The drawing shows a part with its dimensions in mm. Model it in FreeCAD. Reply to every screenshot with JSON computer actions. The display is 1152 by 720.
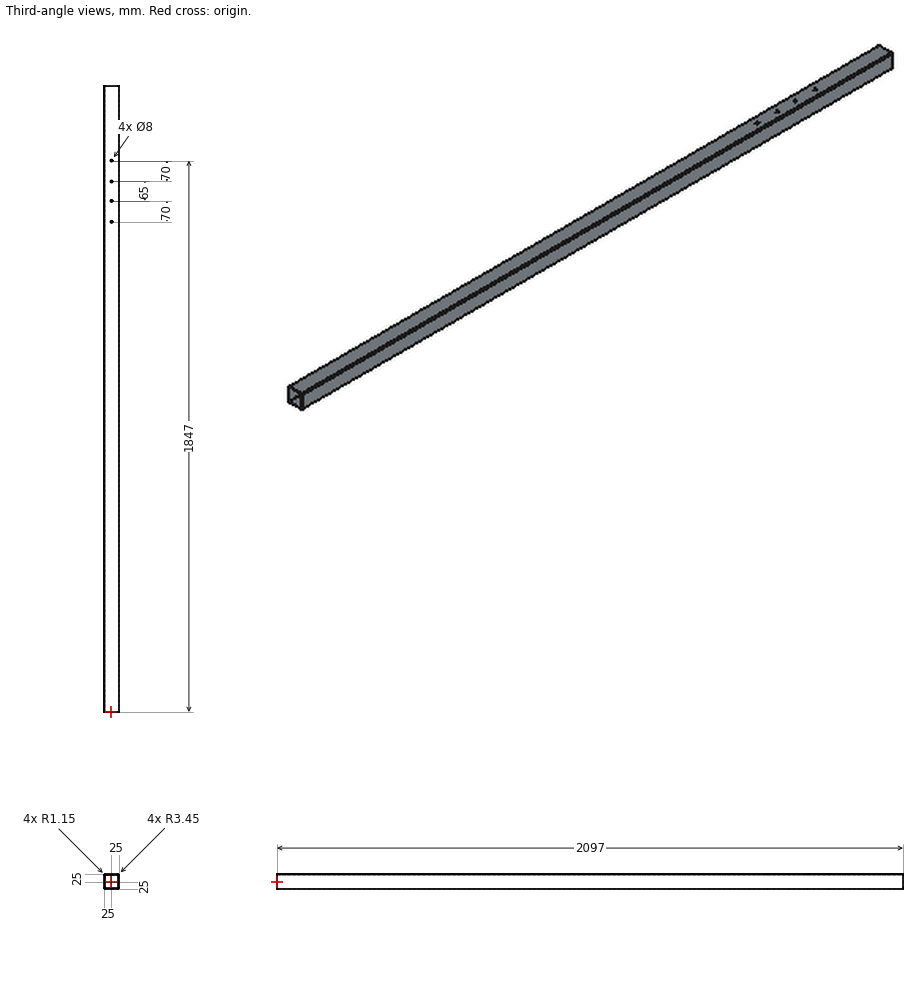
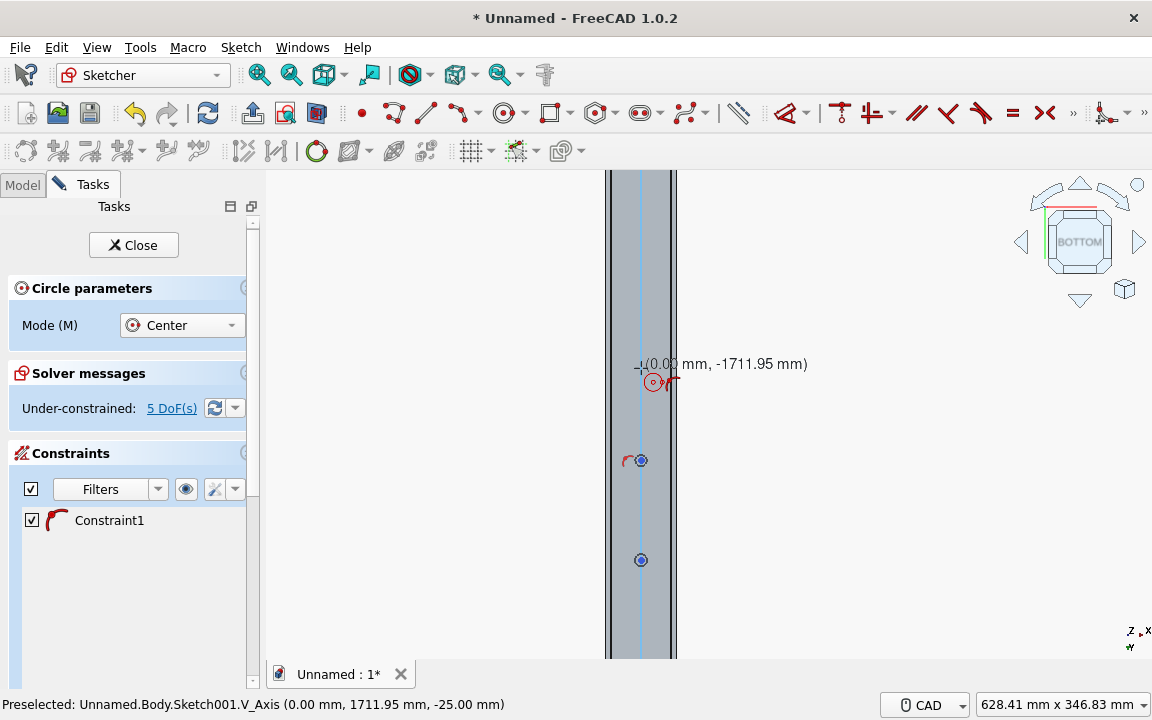
{"action": "left_click", "coordinate": [641, 369]}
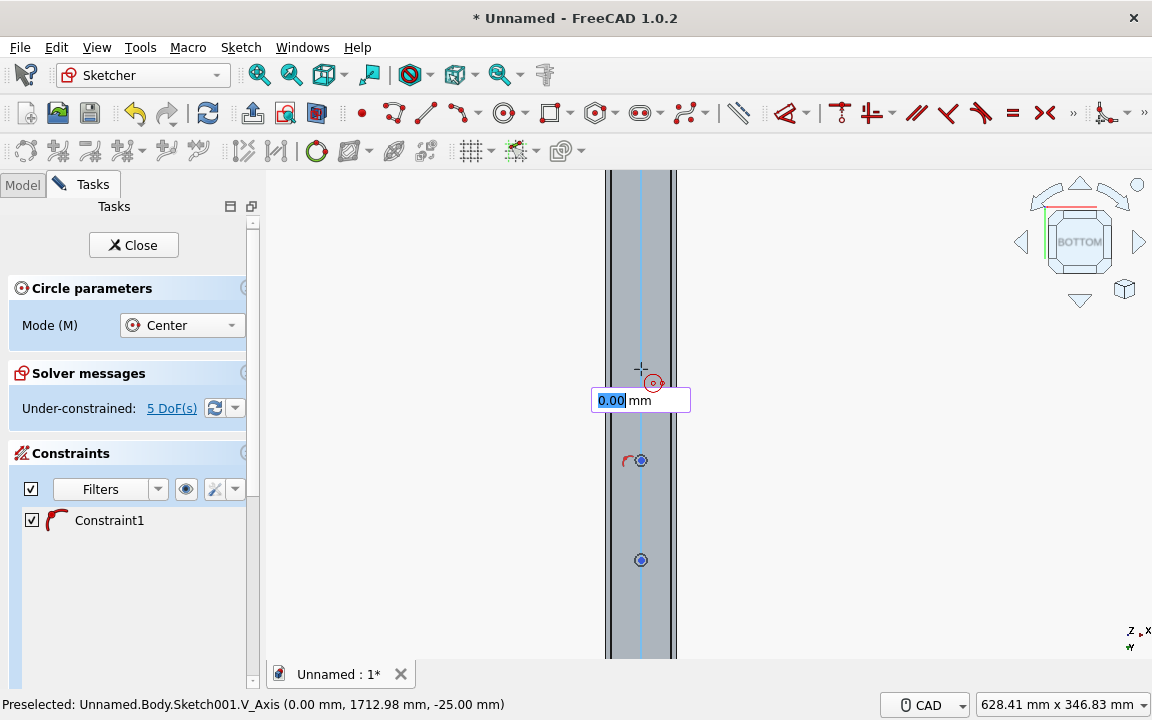
{"action": "scroll", "coordinate": [646, 367], "scroll_direction": "up", "scroll_amount": 6}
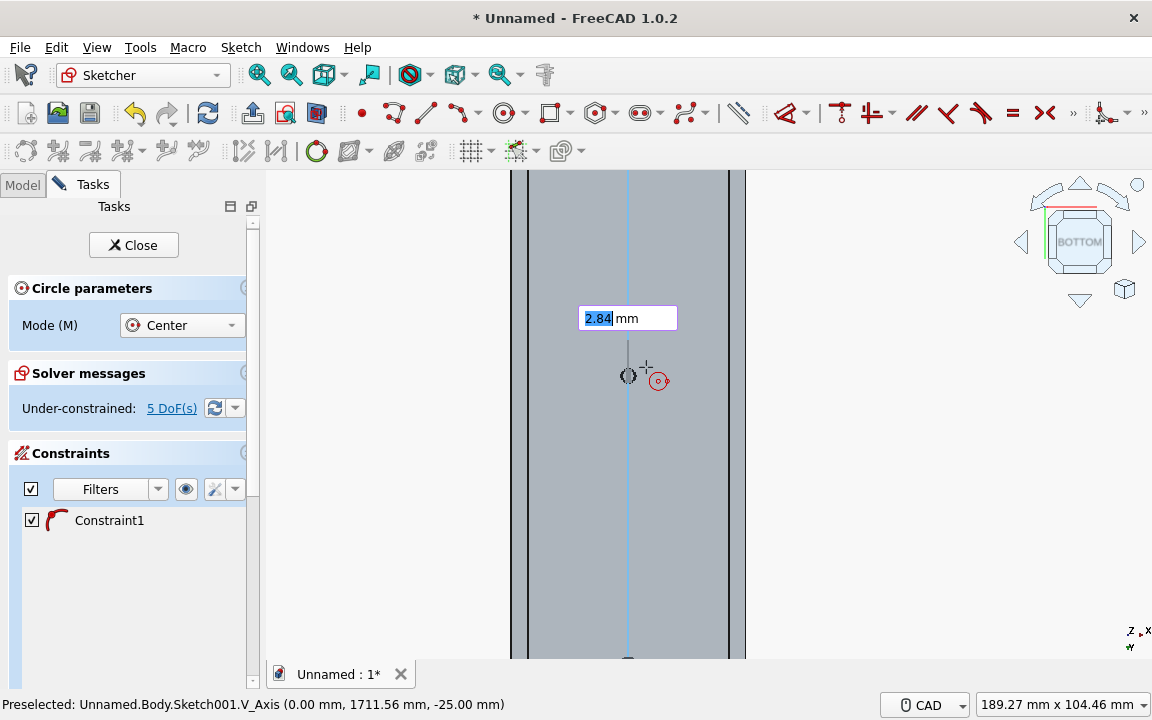
{"action": "left_click", "coordinate": [646, 365]}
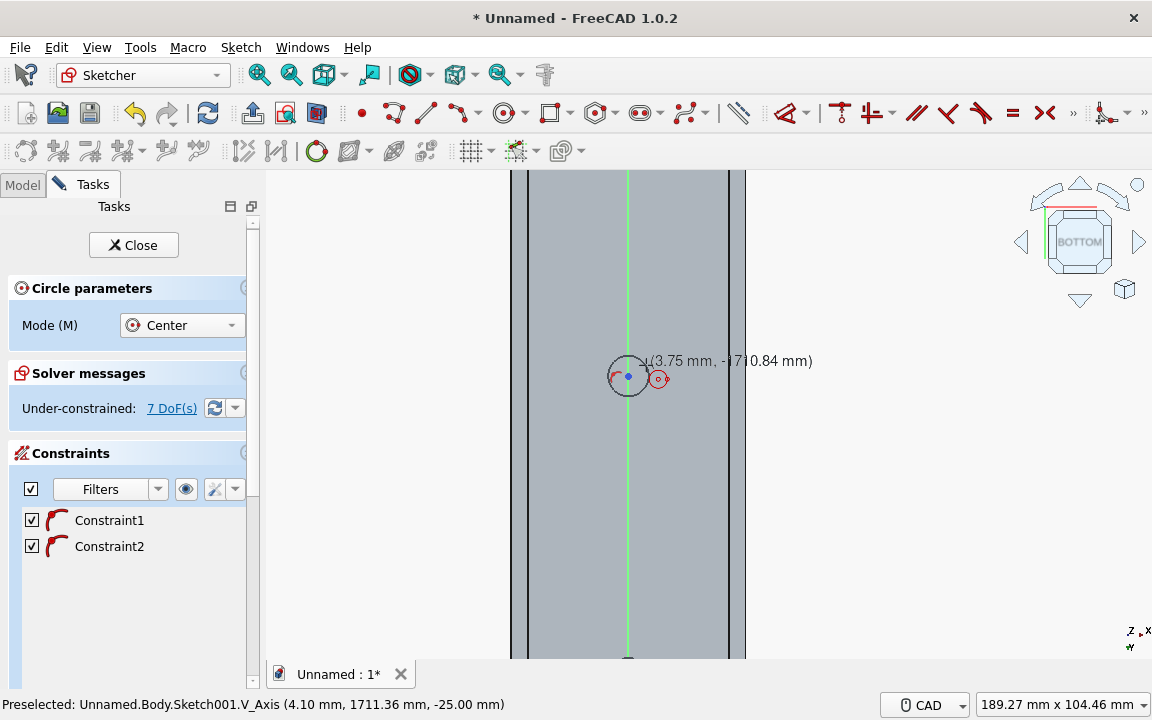
{"action": "scroll", "coordinate": [646, 367], "scroll_direction": "down", "scroll_amount": 6}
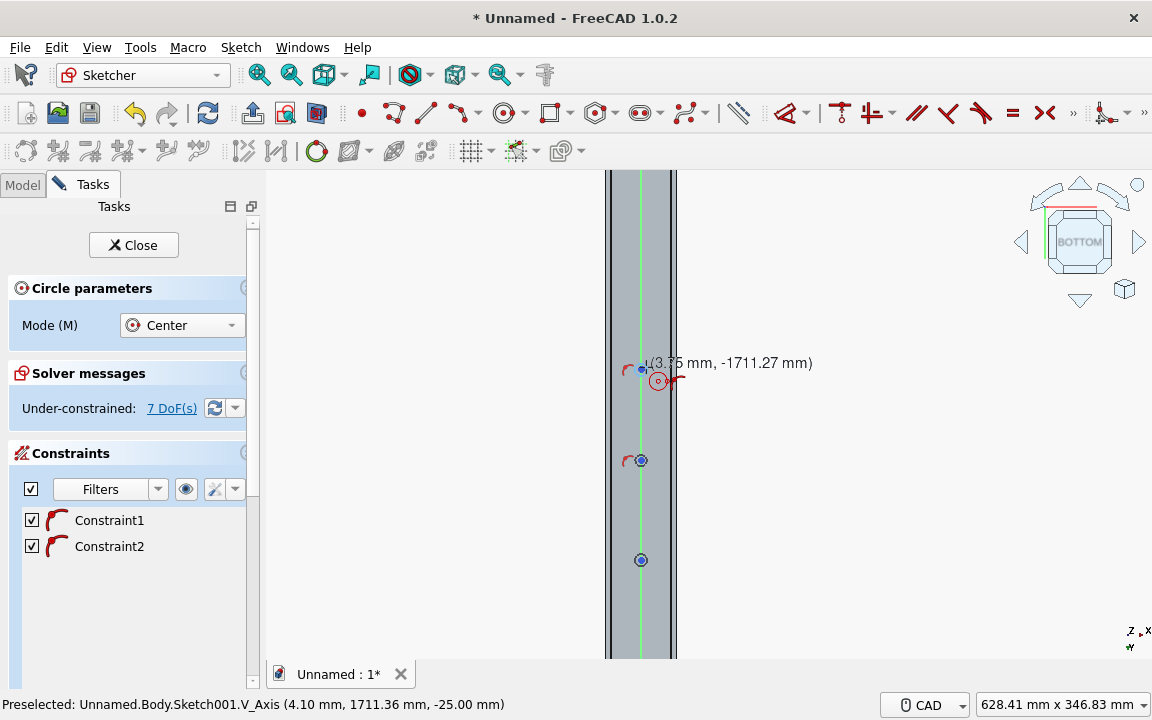
{"action": "scroll", "coordinate": [641, 270], "scroll_direction": "up", "scroll_amount": 7}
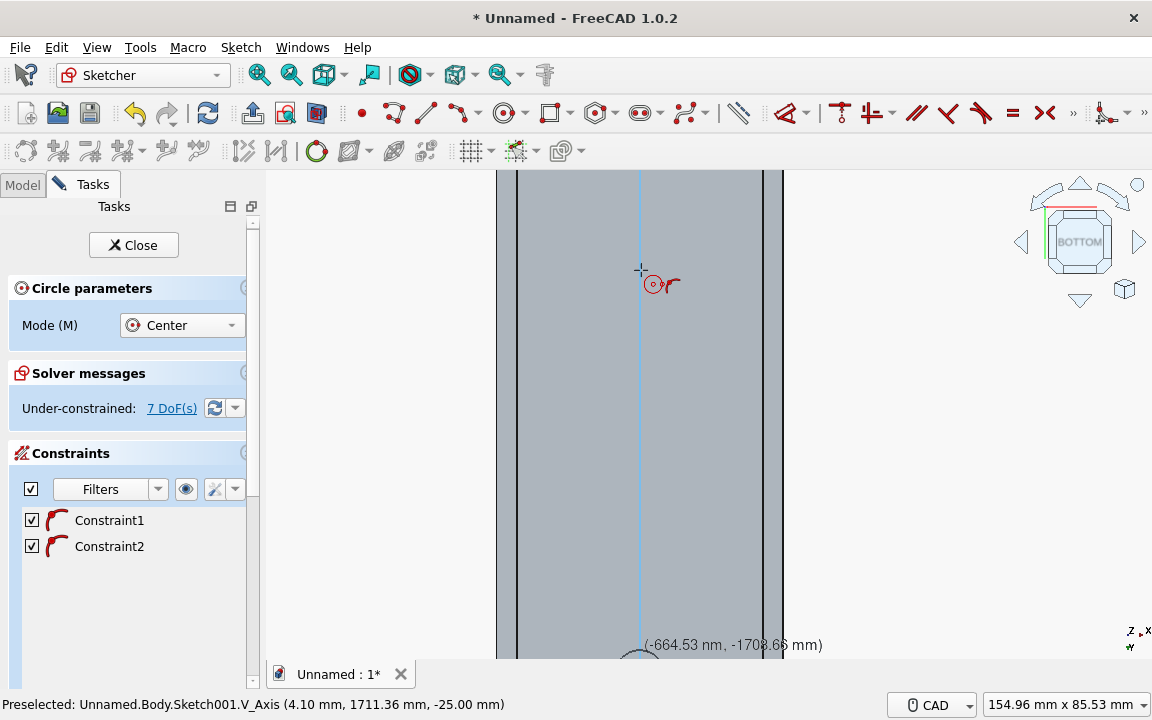
{"action": "scroll", "coordinate": [641, 270], "scroll_direction": "down", "scroll_amount": 7}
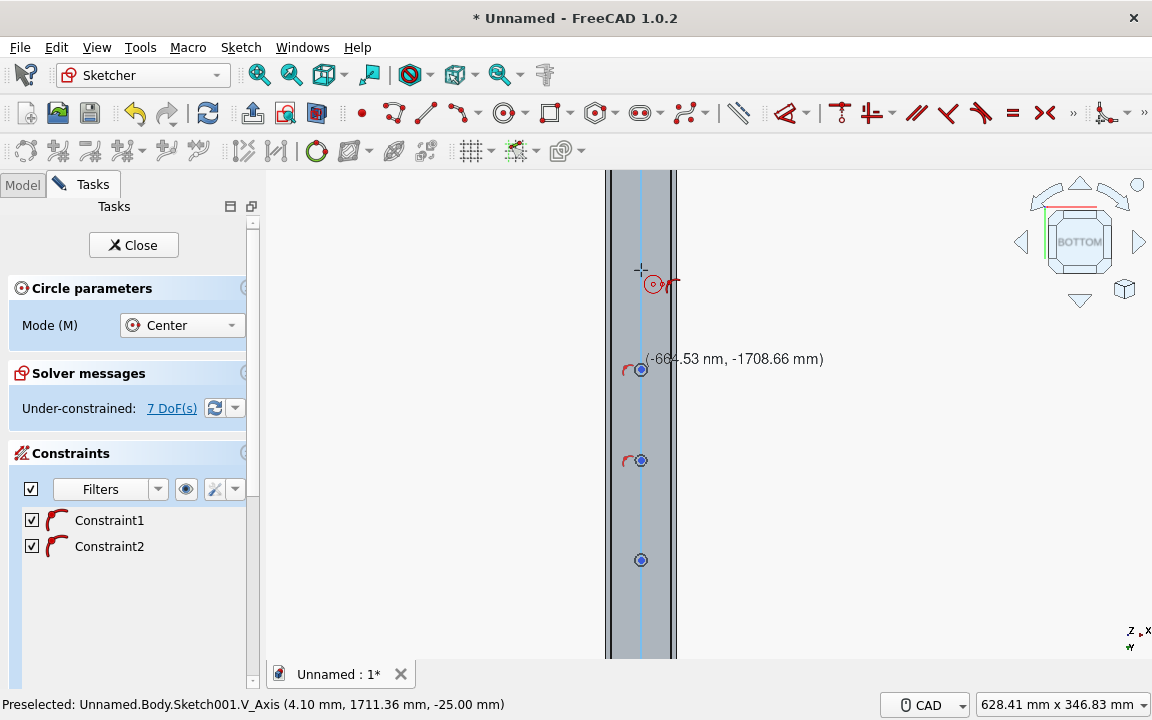
{"action": "left_click", "coordinate": [641, 270]}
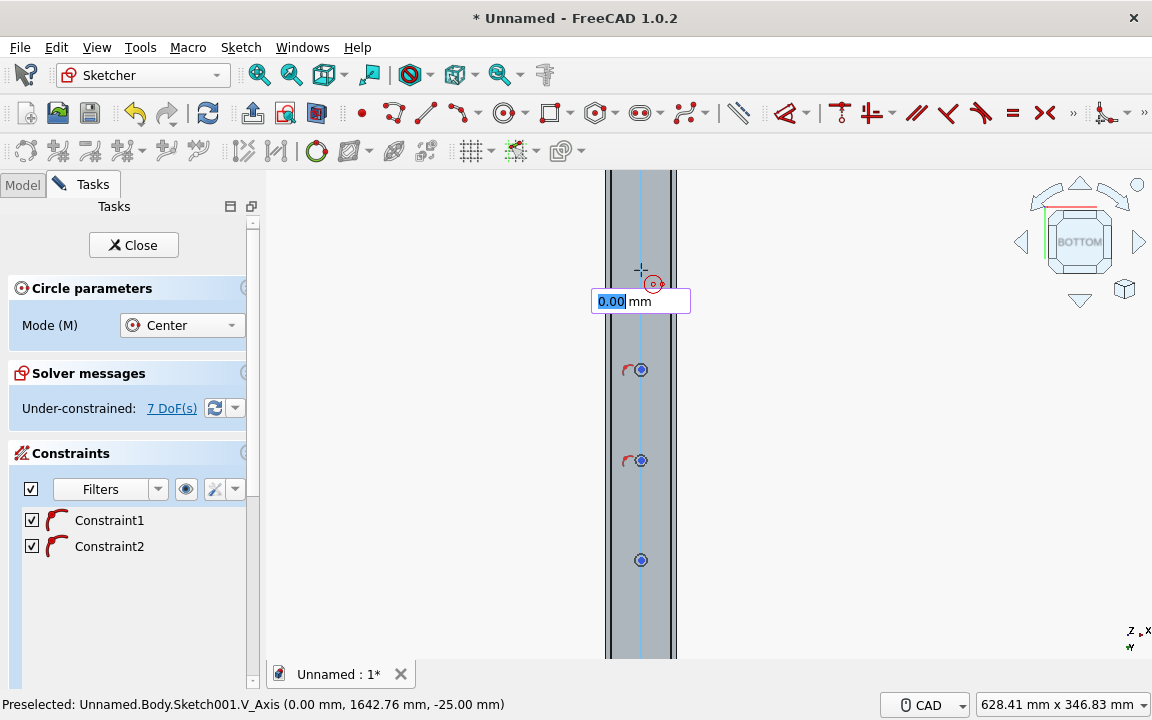
{"action": "scroll", "coordinate": [646, 268], "scroll_direction": "up", "scroll_amount": 6}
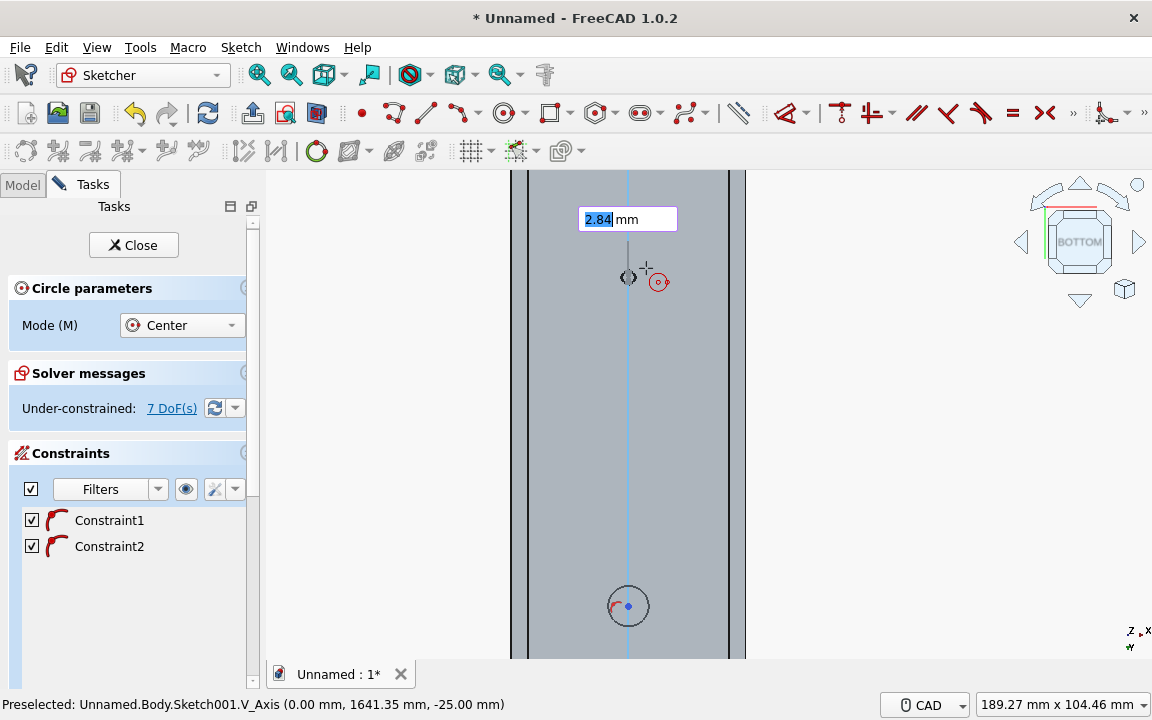
{"action": "left_click", "coordinate": [646, 268]}
{"action": "key", "text": "Escape"}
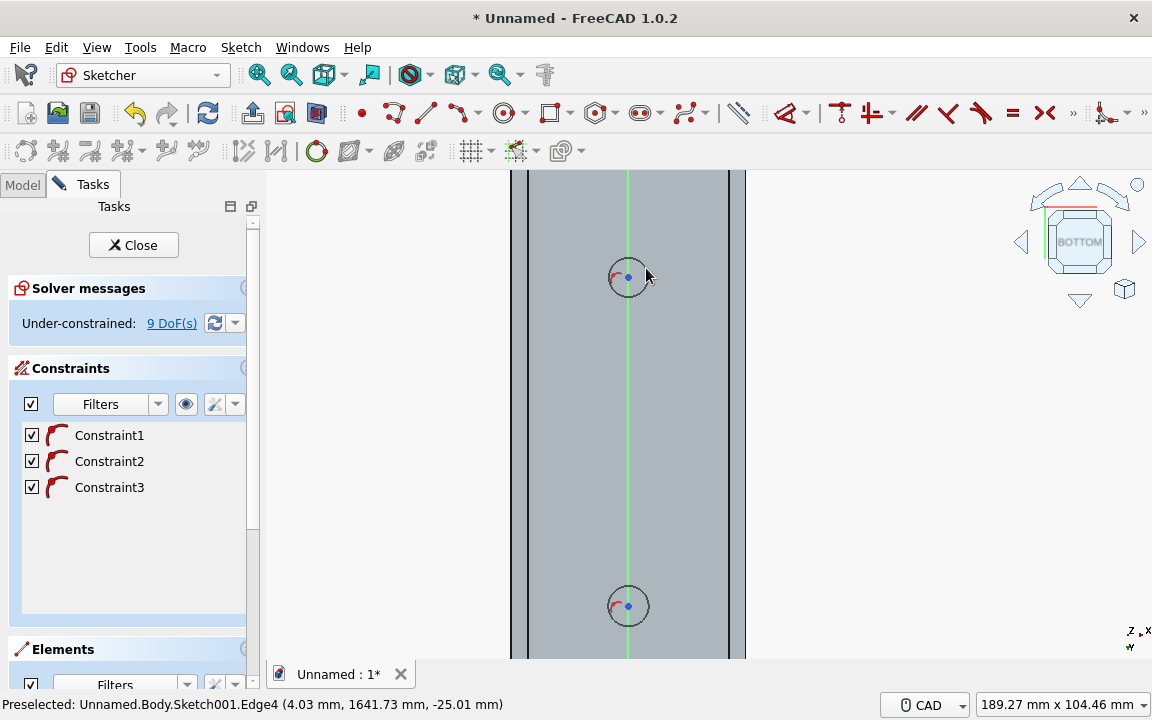
{"action": "scroll", "coordinate": [646, 268], "scroll_direction": "down", "scroll_amount": 6}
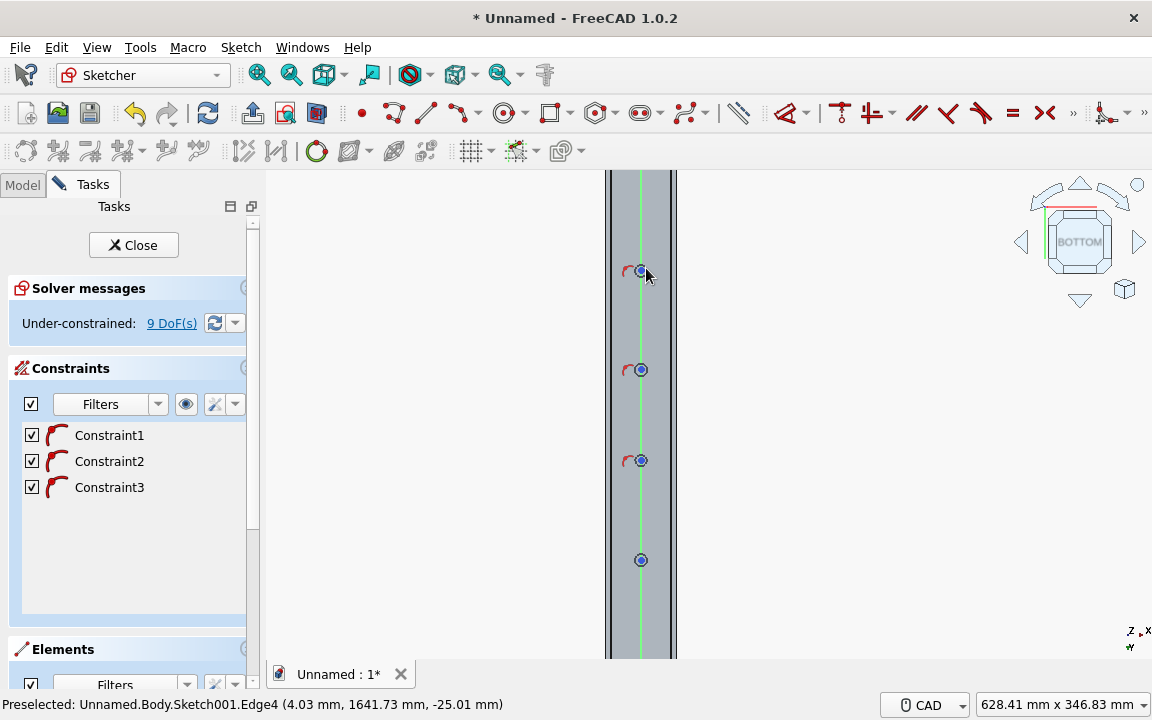
{"action": "scroll", "coordinate": [645, 556], "scroll_direction": "up", "scroll_amount": 6}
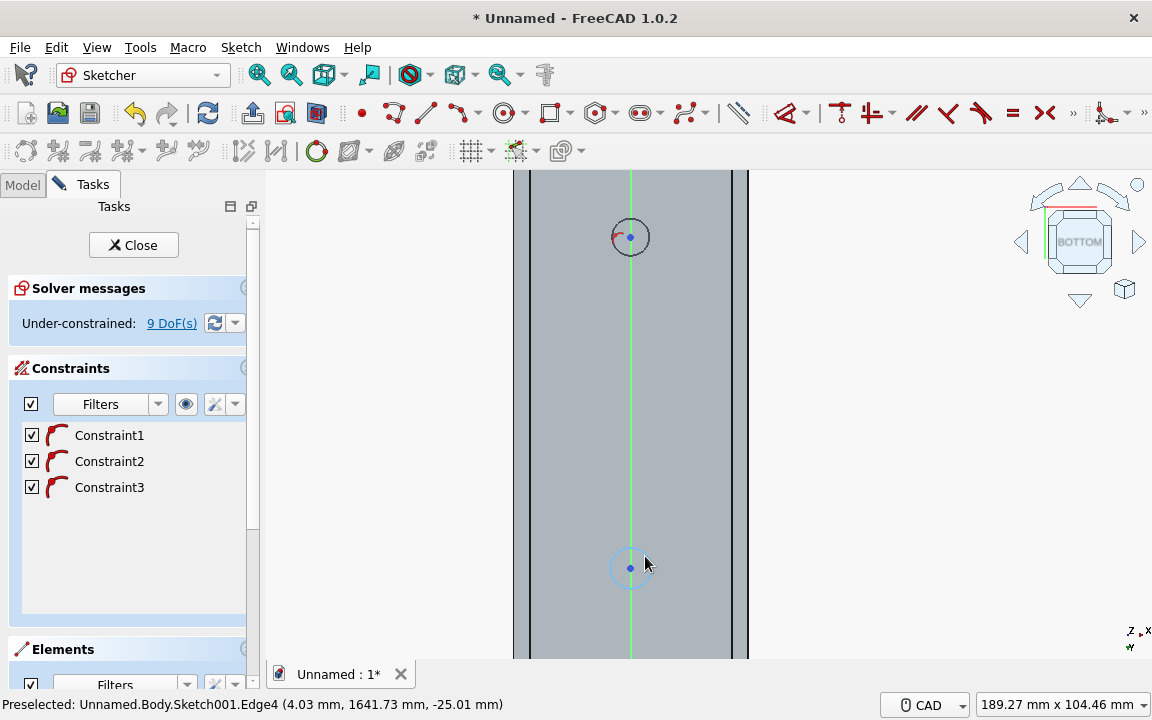
{"action": "left_click", "coordinate": [645, 554]}